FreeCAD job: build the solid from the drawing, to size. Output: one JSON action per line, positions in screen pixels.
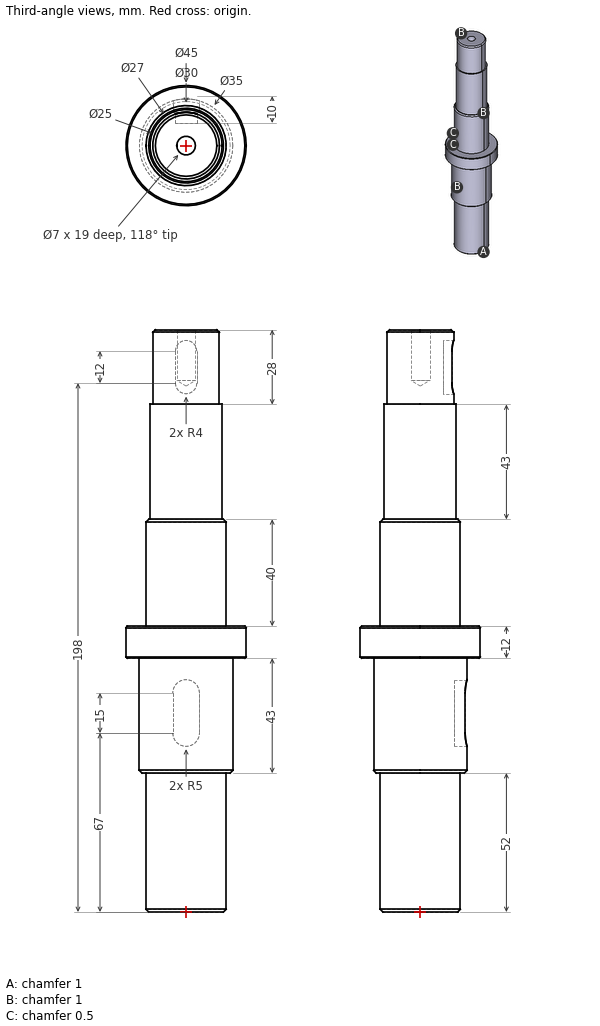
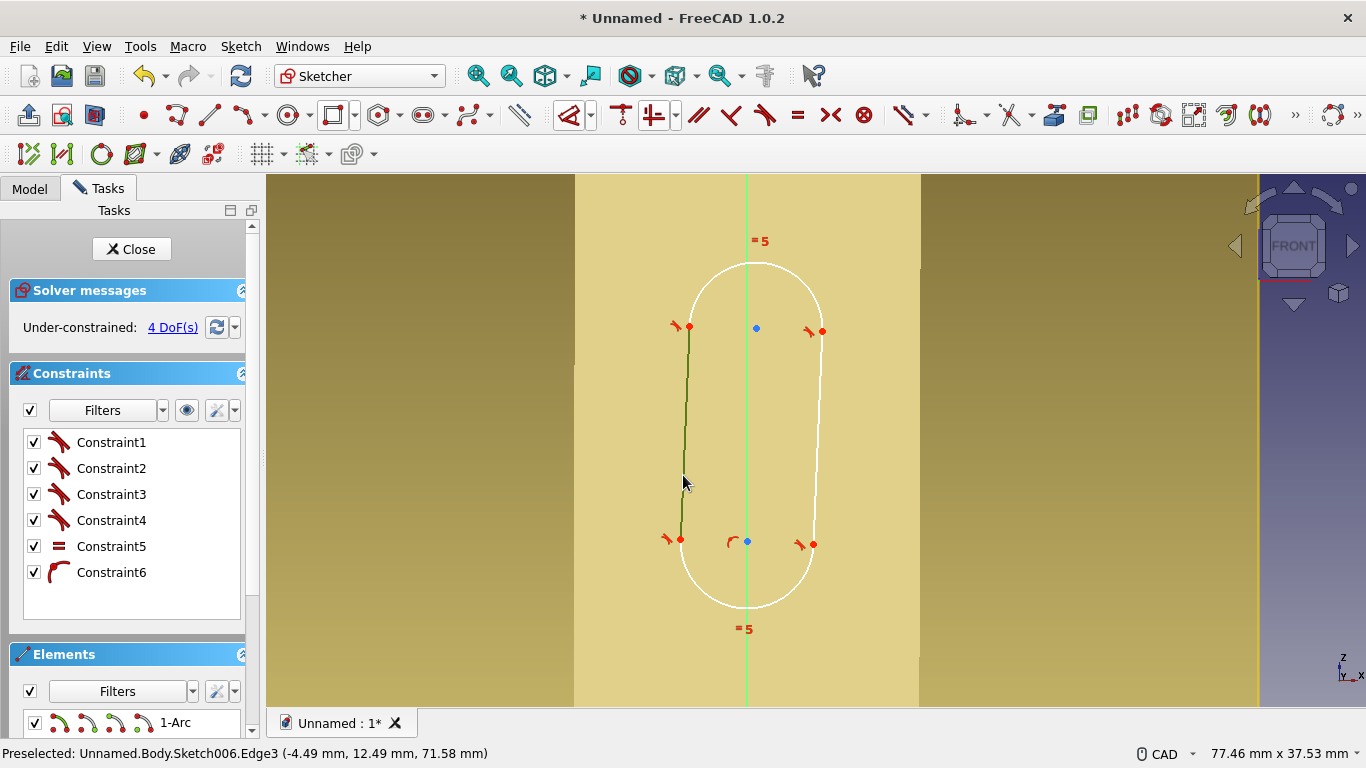
{"action": "key", "text": "v"}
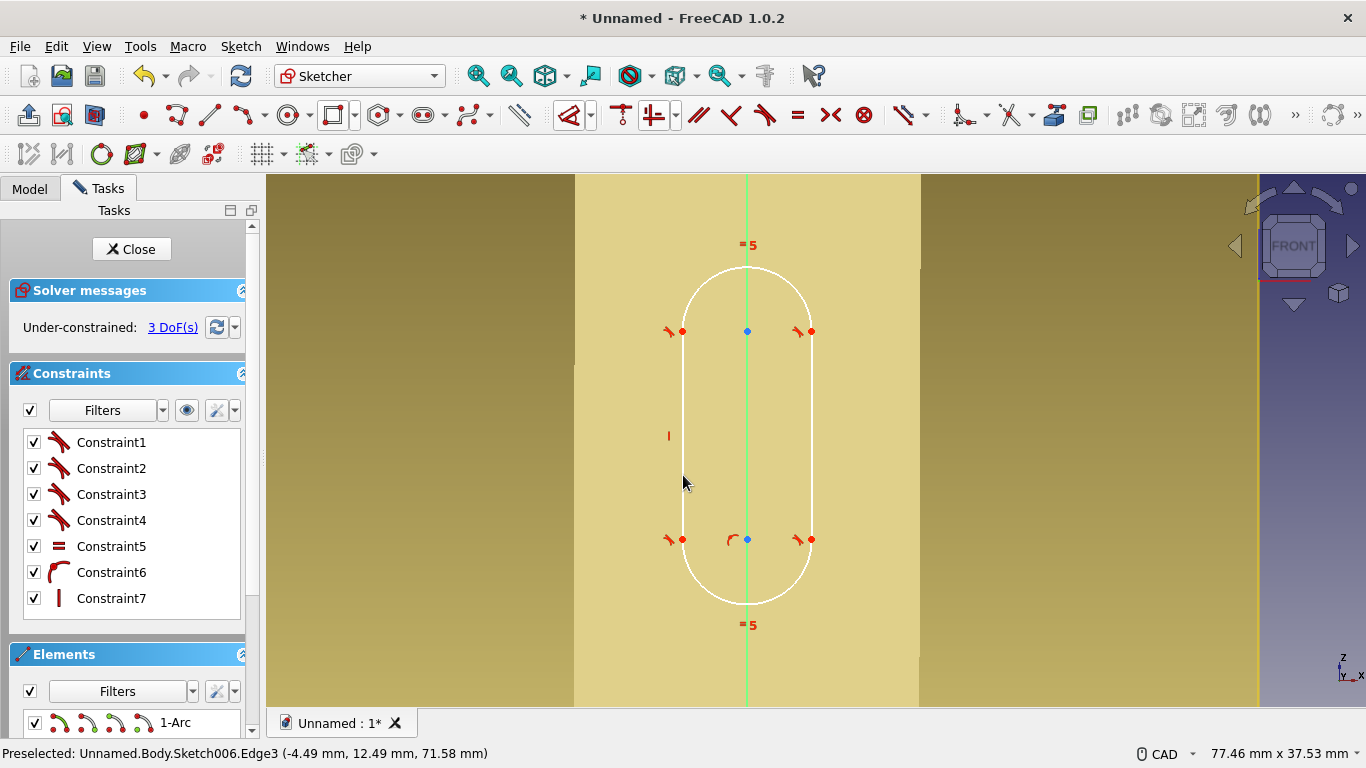
{"action": "left_click", "coordinate": [709, 592]}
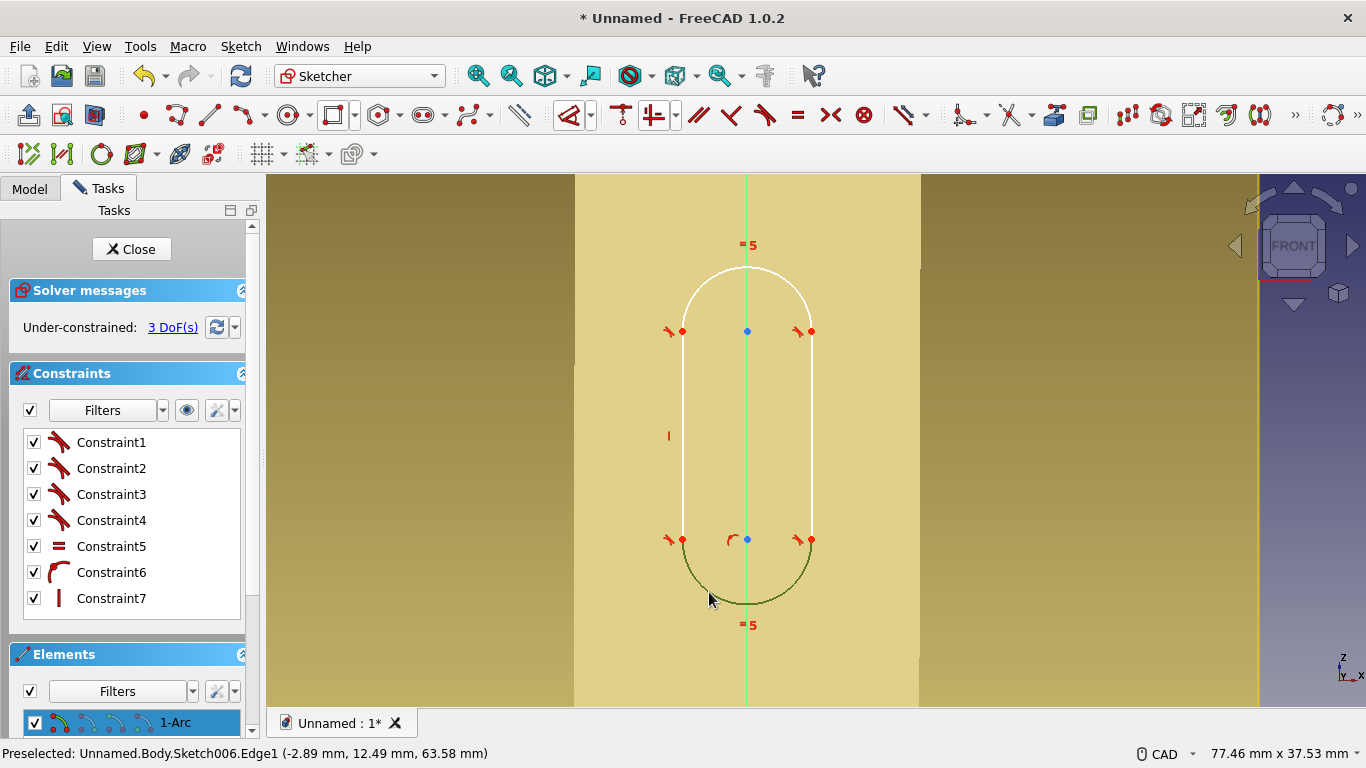
{"action": "key", "text": "k r"}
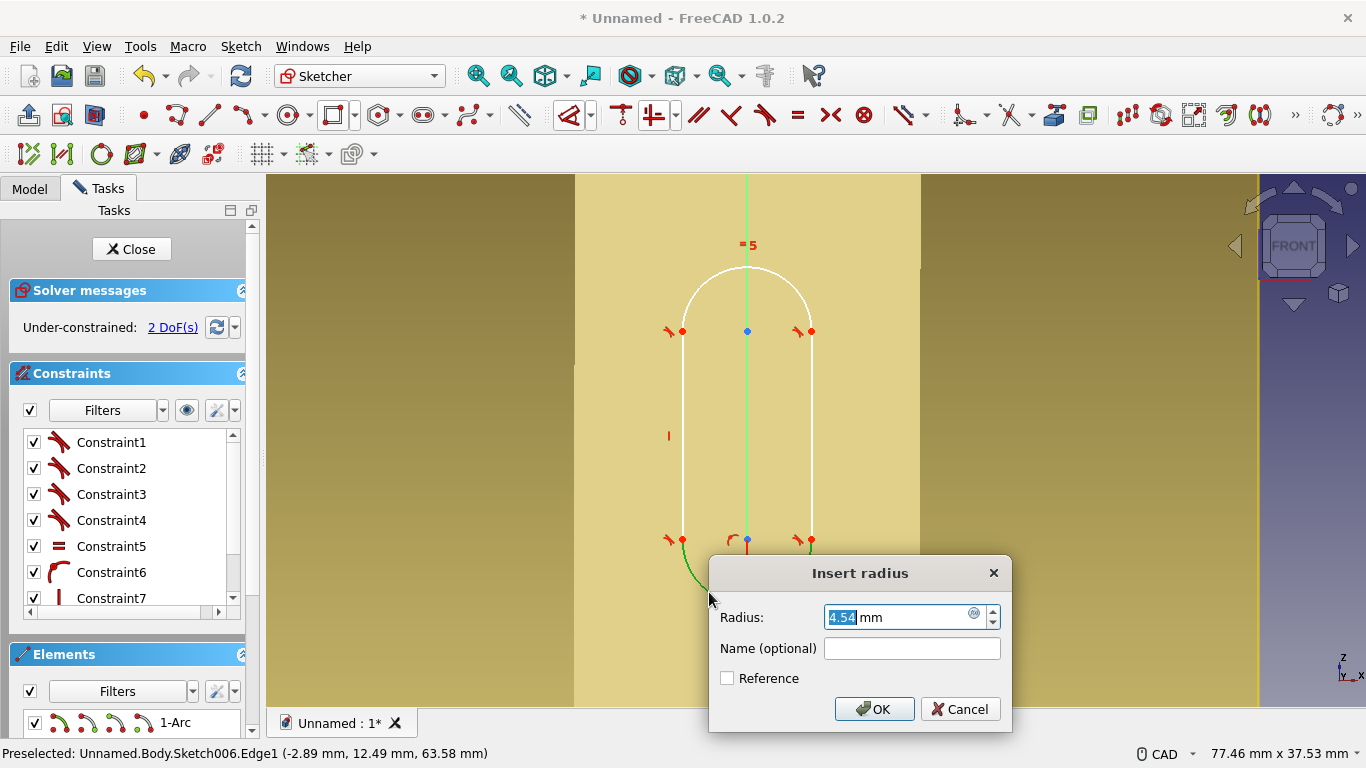
{"action": "type", "text": "5"}
{"action": "key", "text": "Return"}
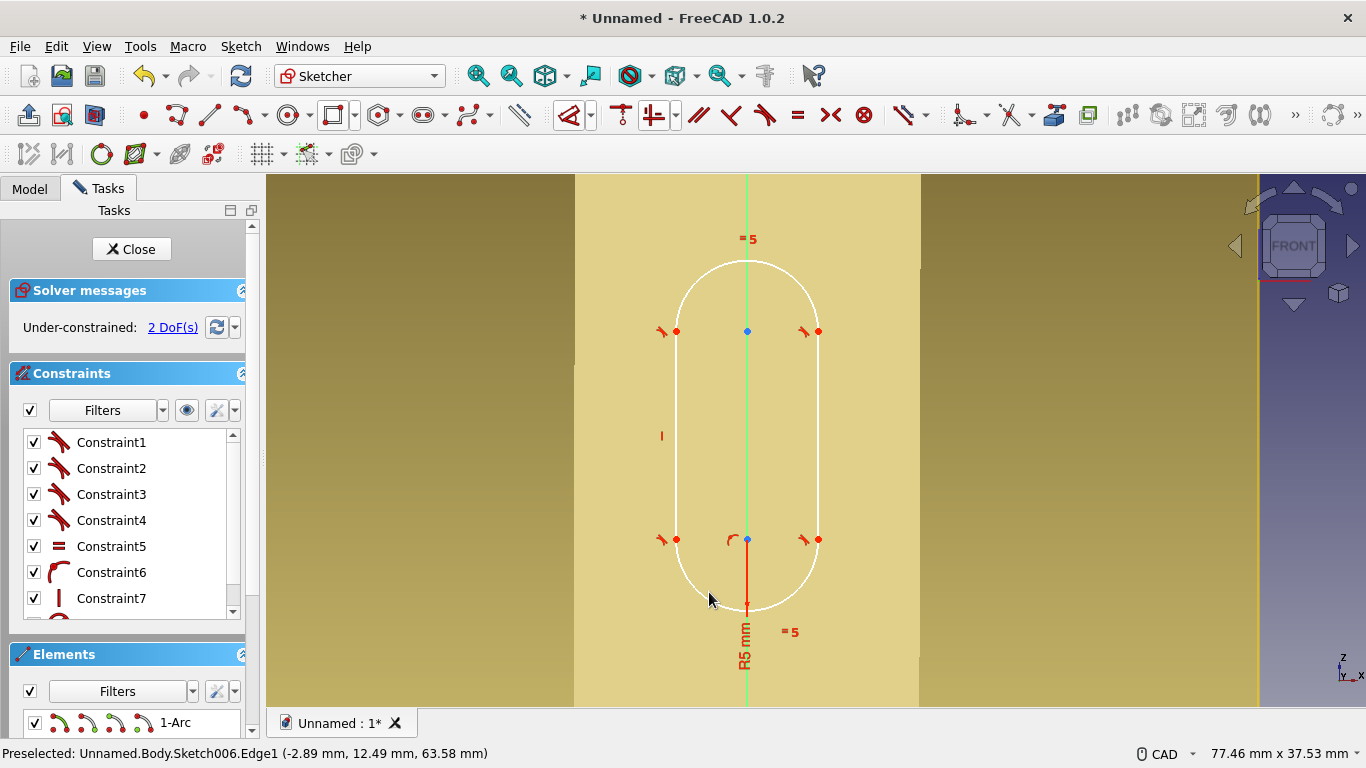
{"action": "left_click", "coordinate": [676, 478]}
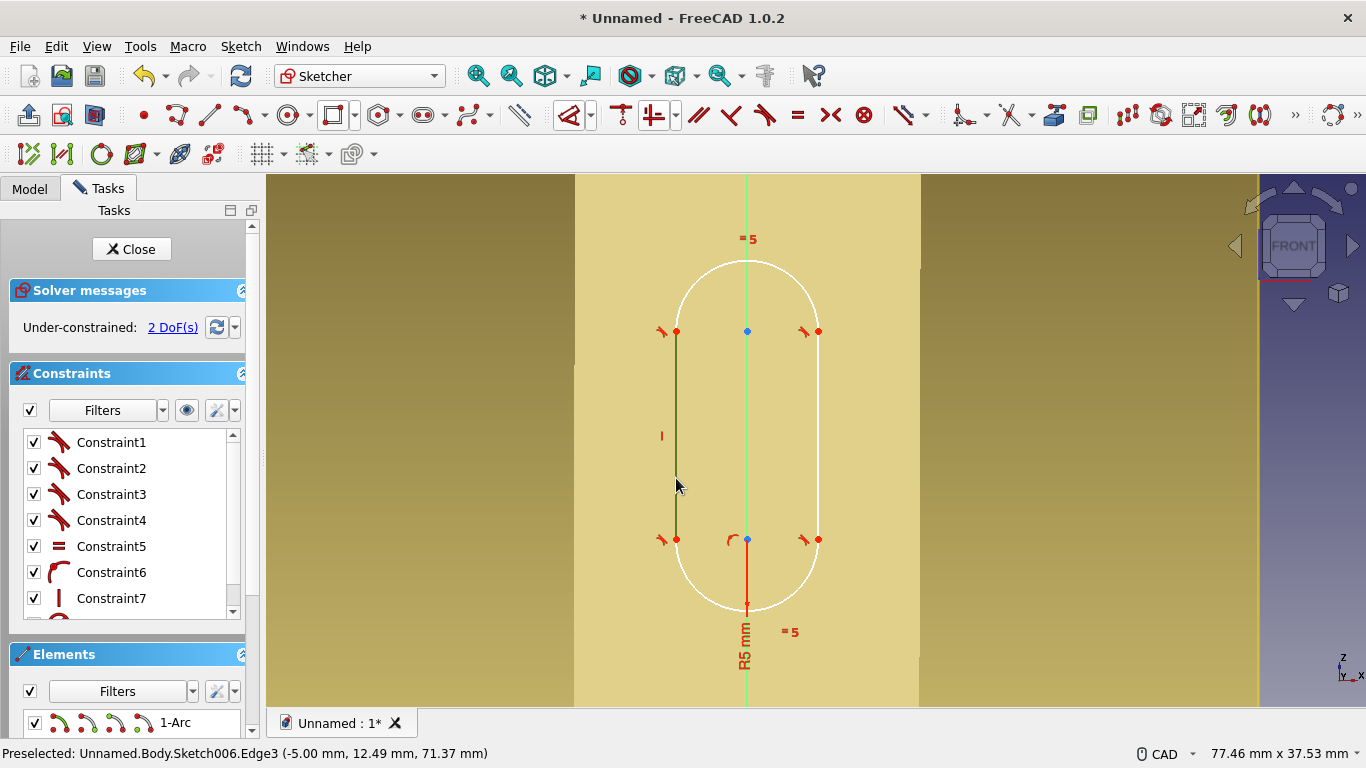
{"action": "key", "text": "i"}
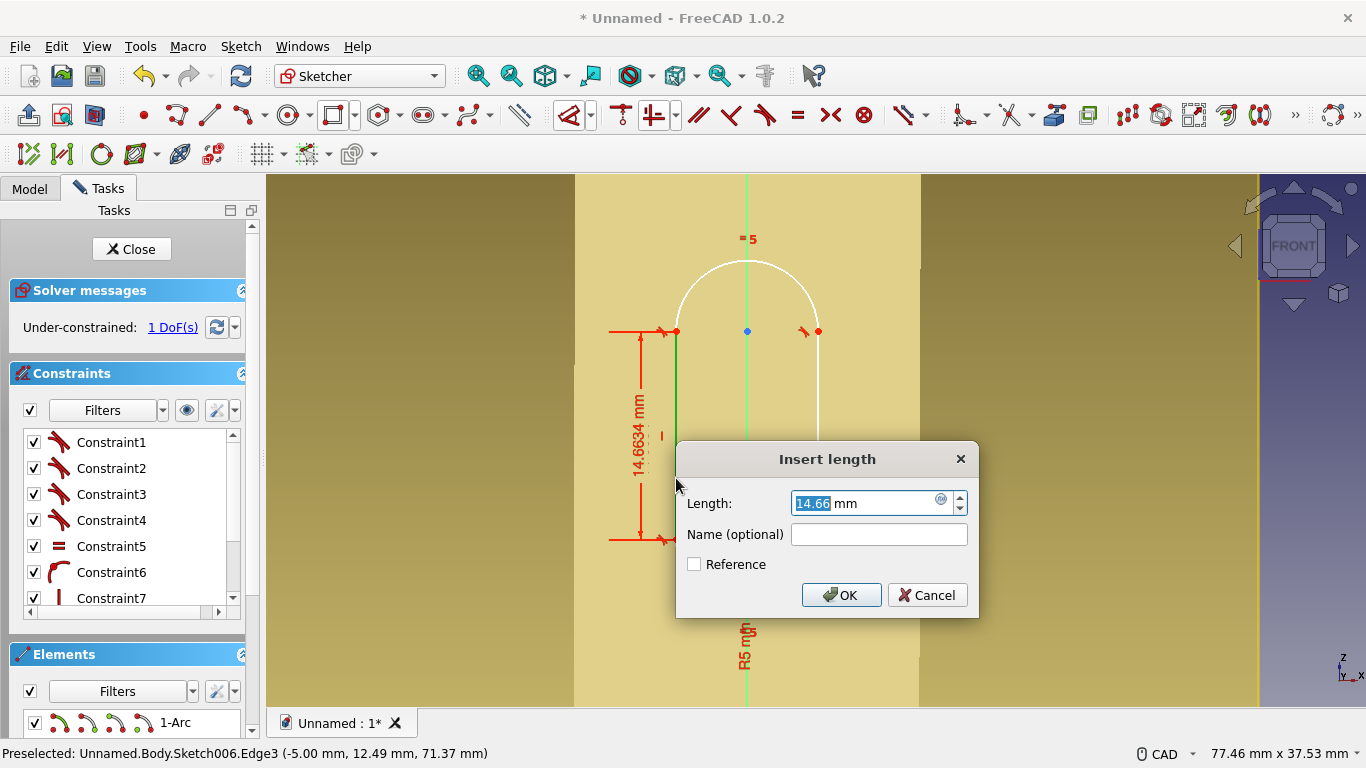
{"action": "type", "text": "15"}
{"action": "key", "text": "Return"}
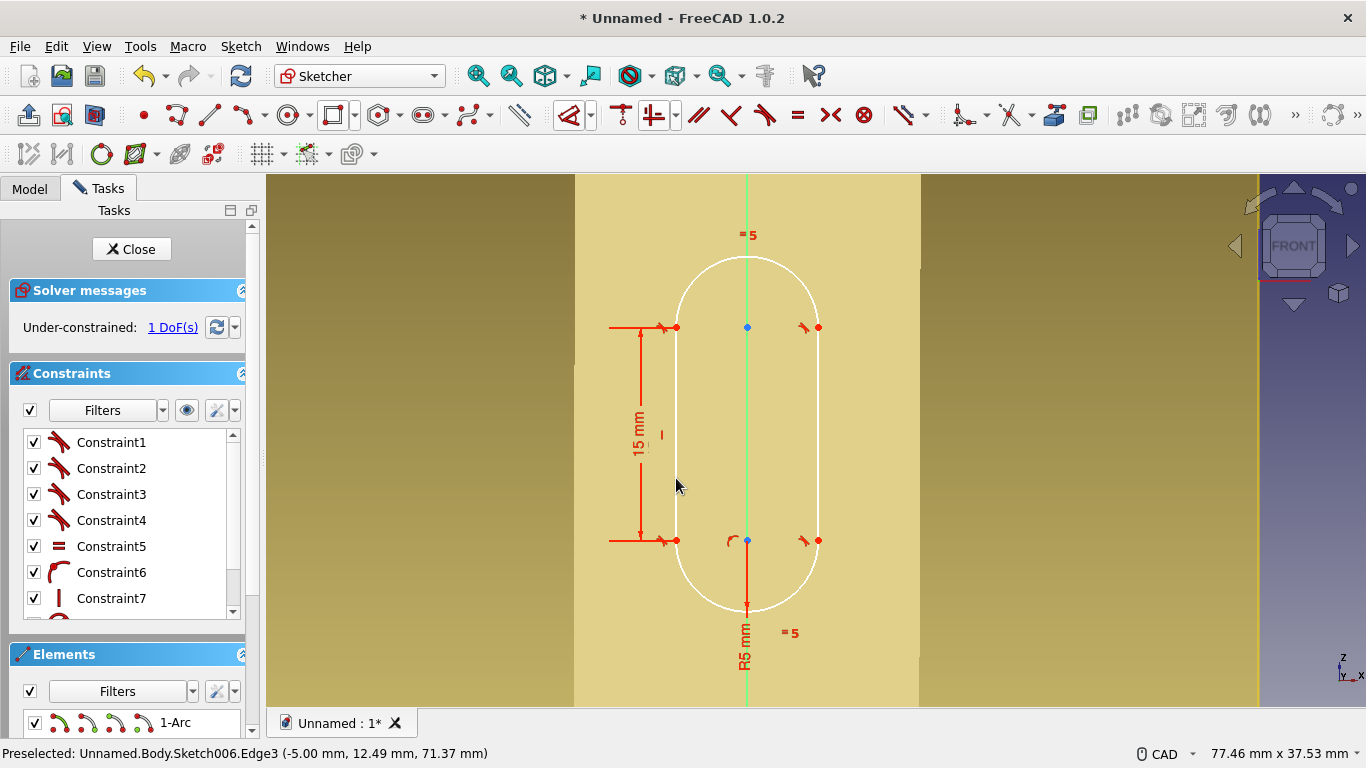
{"action": "left_click", "coordinate": [676, 541]}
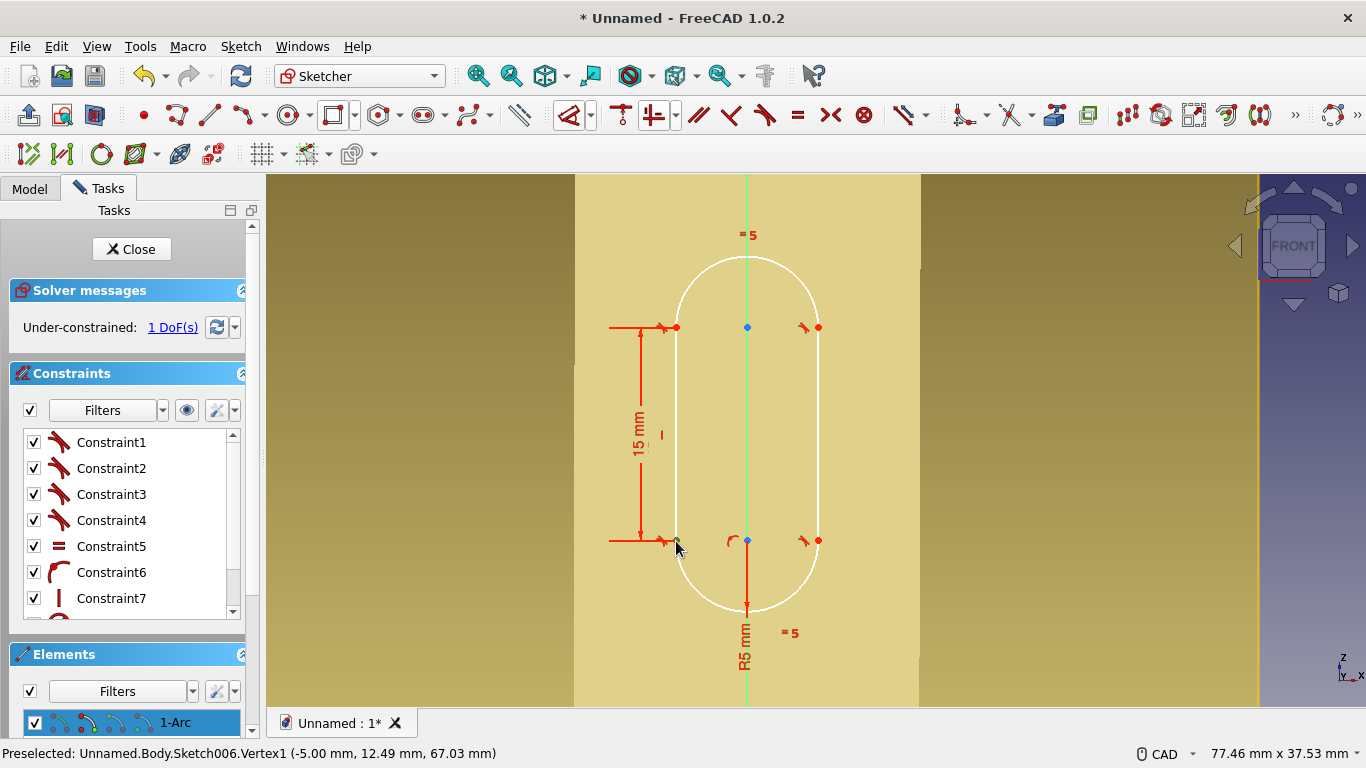
{"action": "key", "text": "i"}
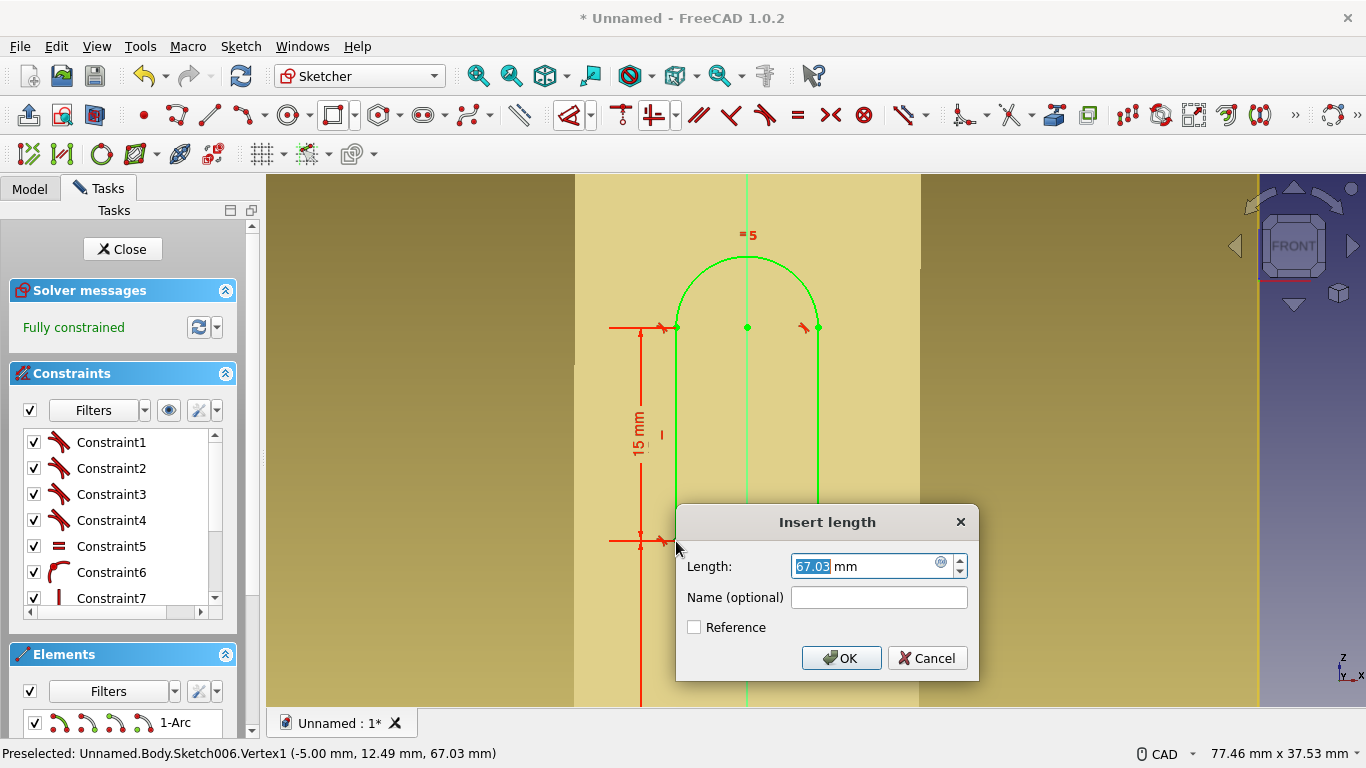
{"action": "type", "text": "67"}
{"action": "key", "text": "Return"}